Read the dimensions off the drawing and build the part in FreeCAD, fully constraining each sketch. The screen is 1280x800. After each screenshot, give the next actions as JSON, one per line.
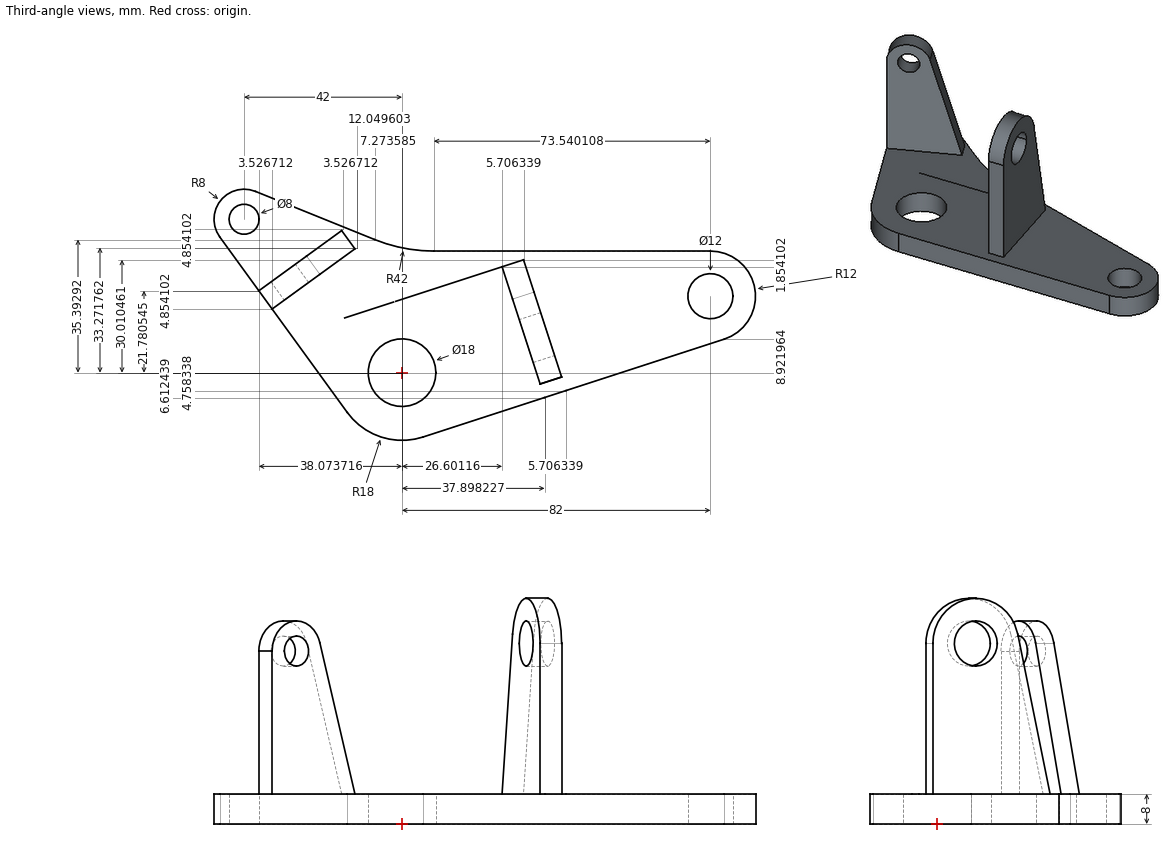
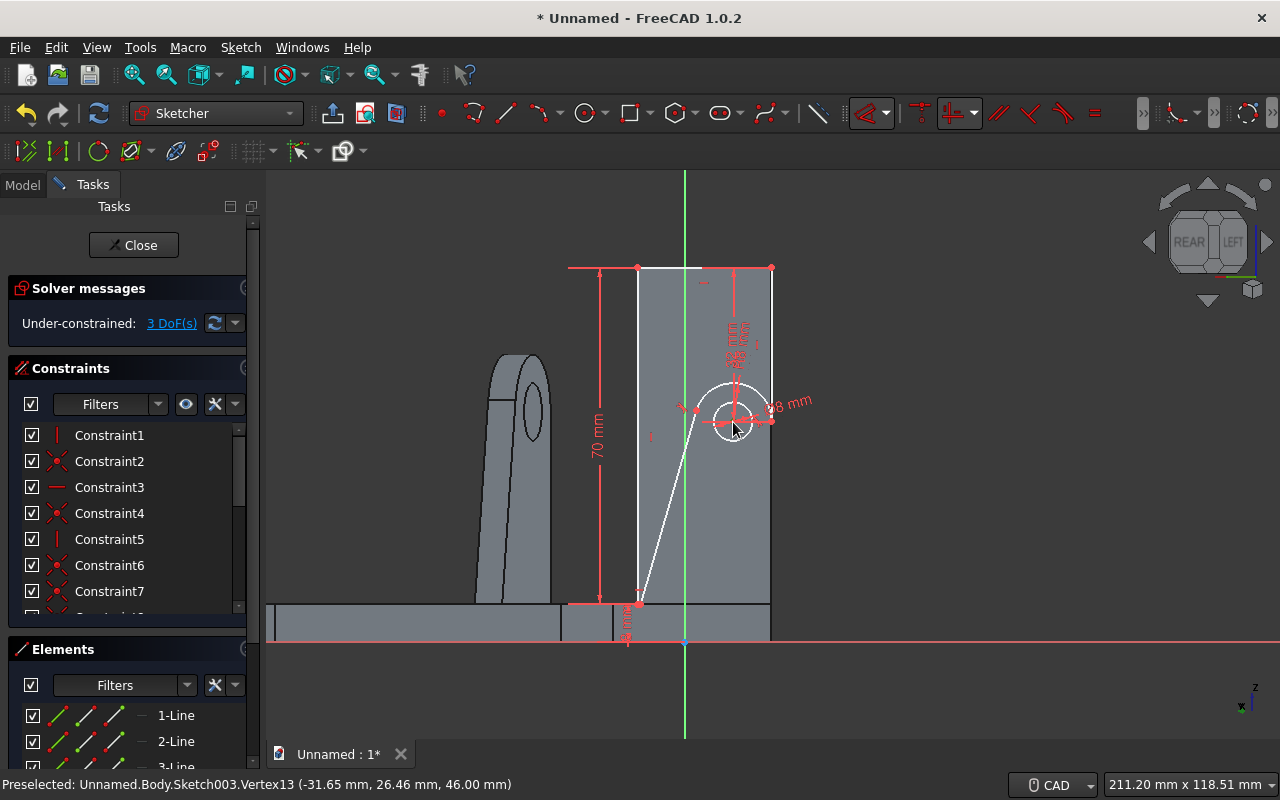
{"action": "key", "text": "l"}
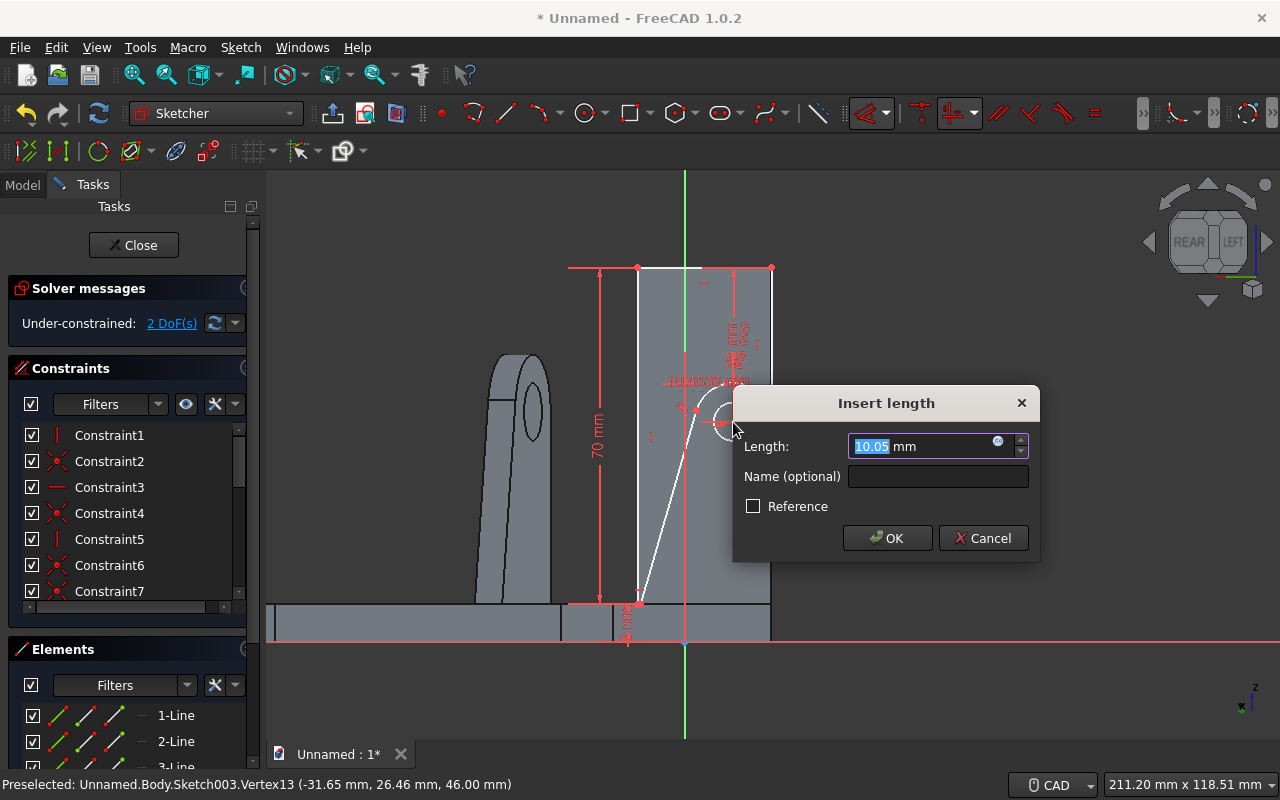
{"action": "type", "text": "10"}
{"action": "key", "text": "Return"}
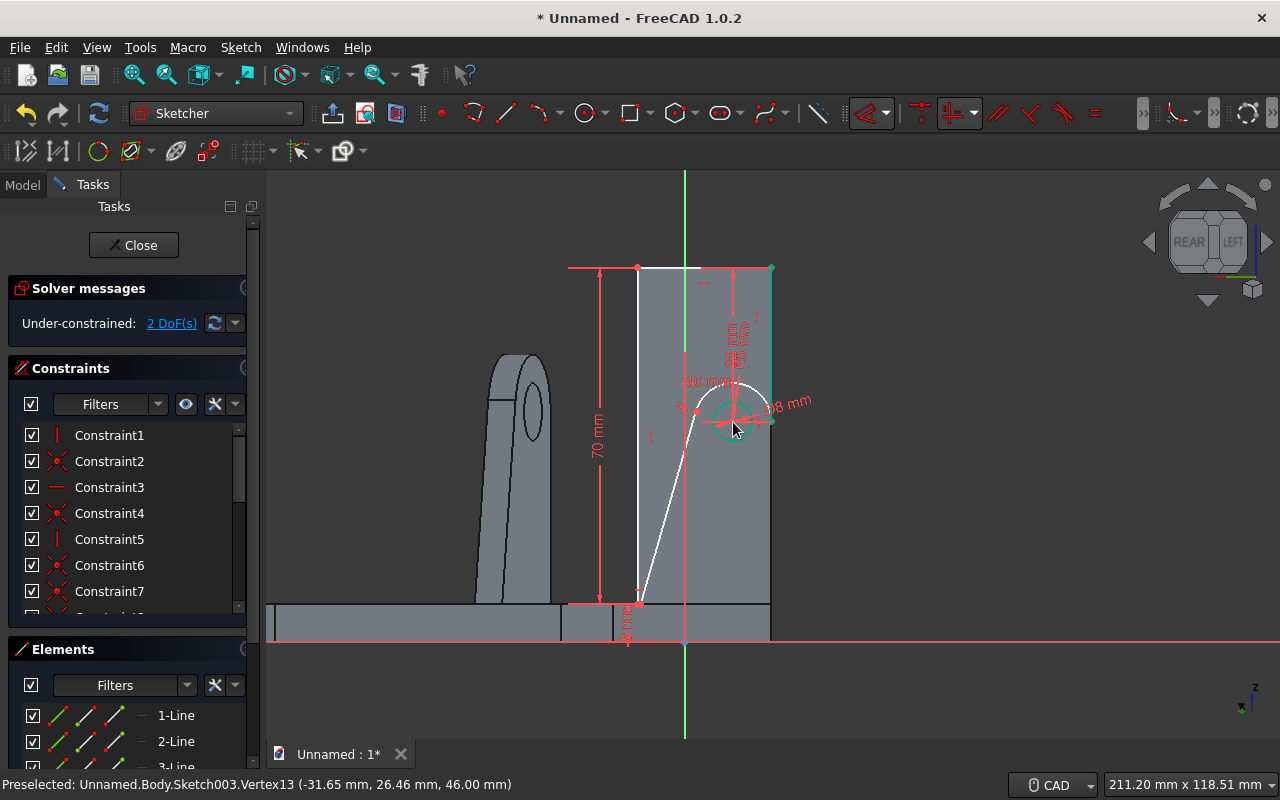
{"action": "scroll", "coordinate": [639, 604], "scroll_direction": "up", "scroll_amount": 14}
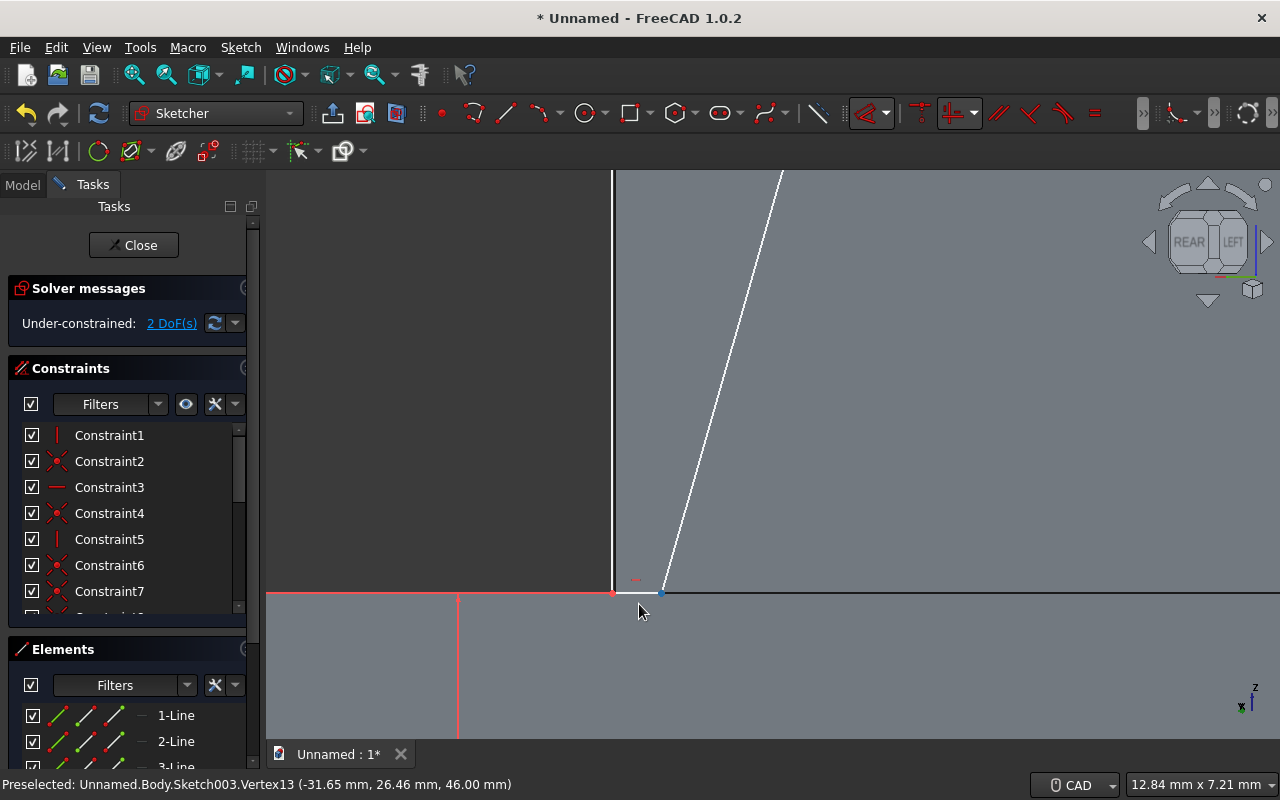
{"action": "left_click", "coordinate": [637, 593]}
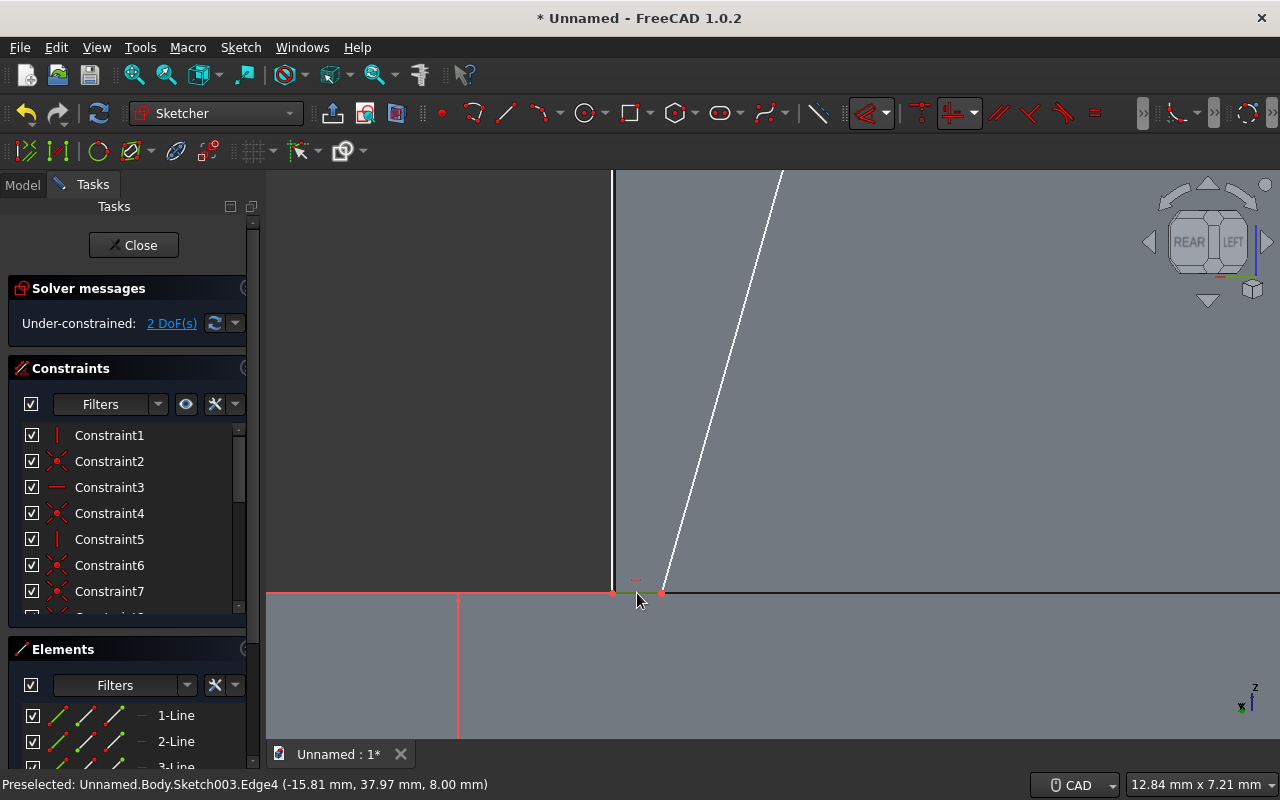
{"action": "key", "text": "l"}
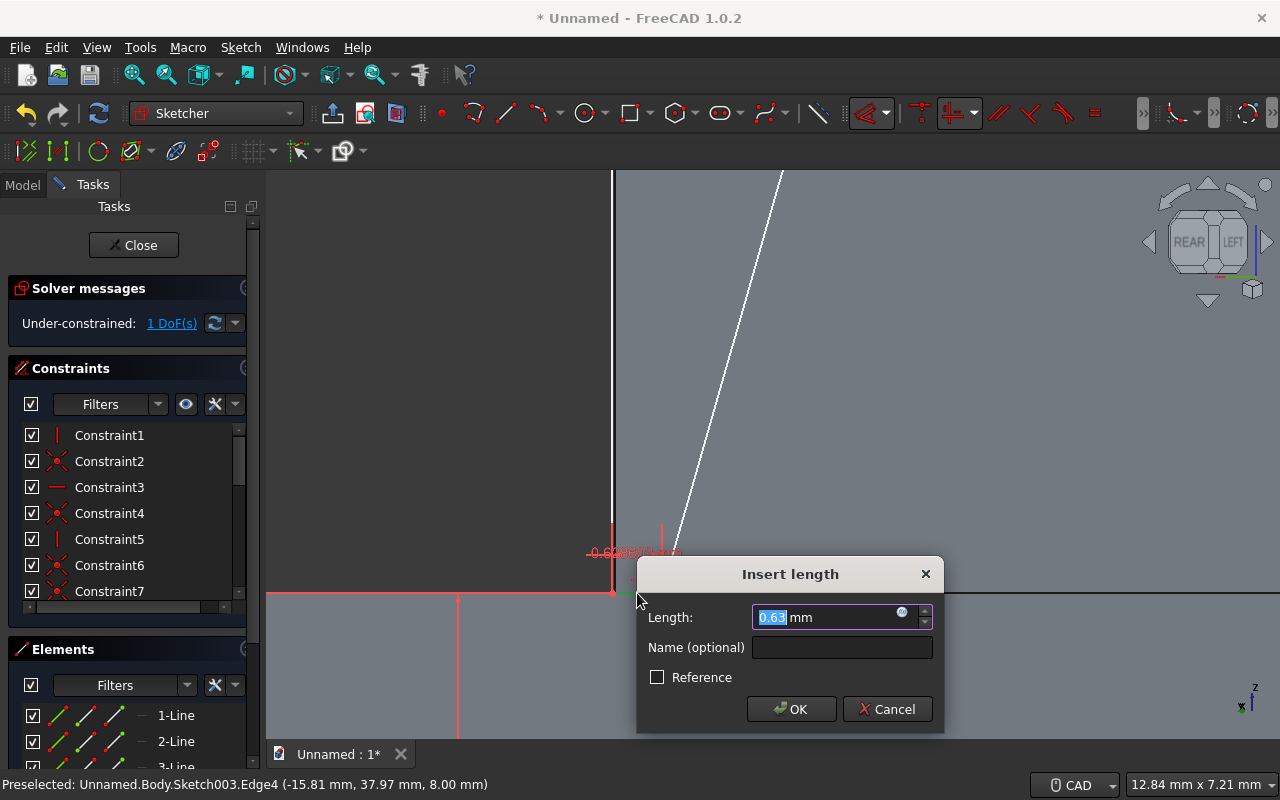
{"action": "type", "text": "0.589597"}
{"action": "key", "text": "Return"}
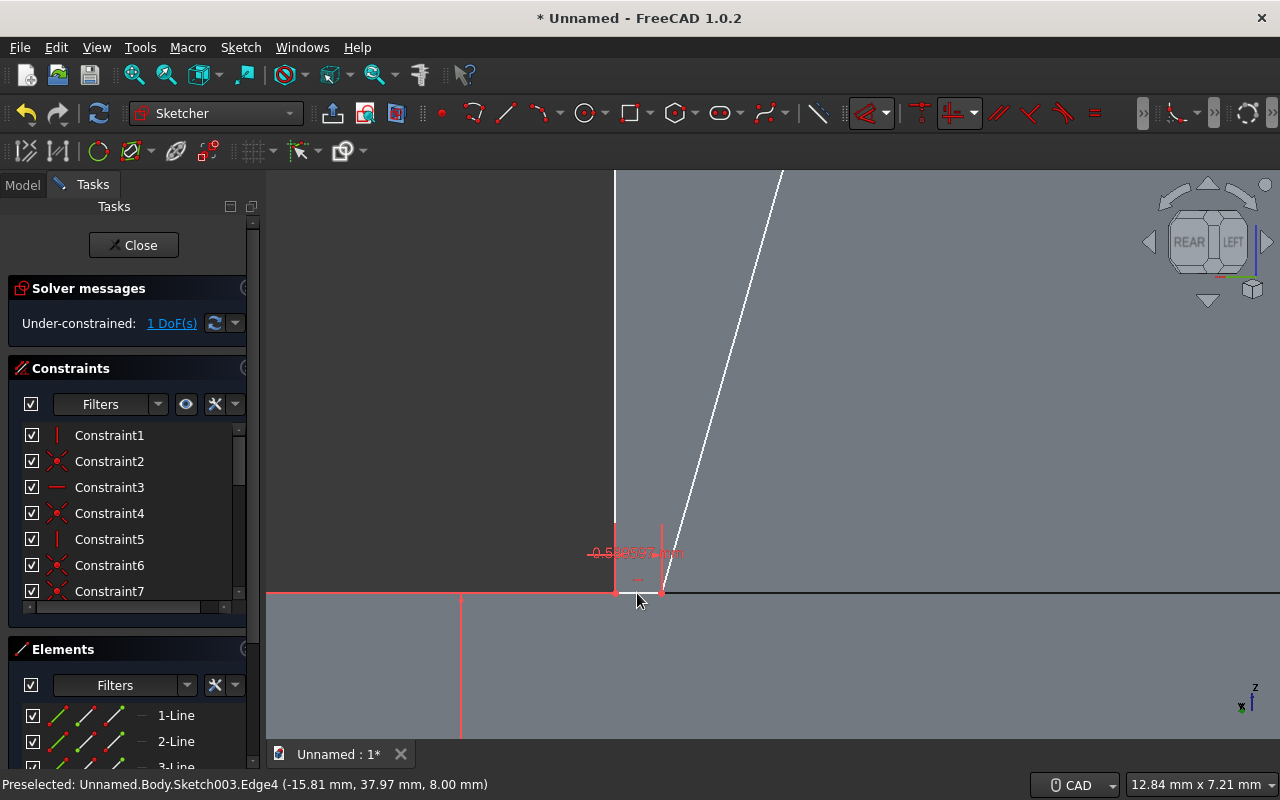
{"action": "scroll", "coordinate": [639, 604], "scroll_direction": "down", "scroll_amount": 14}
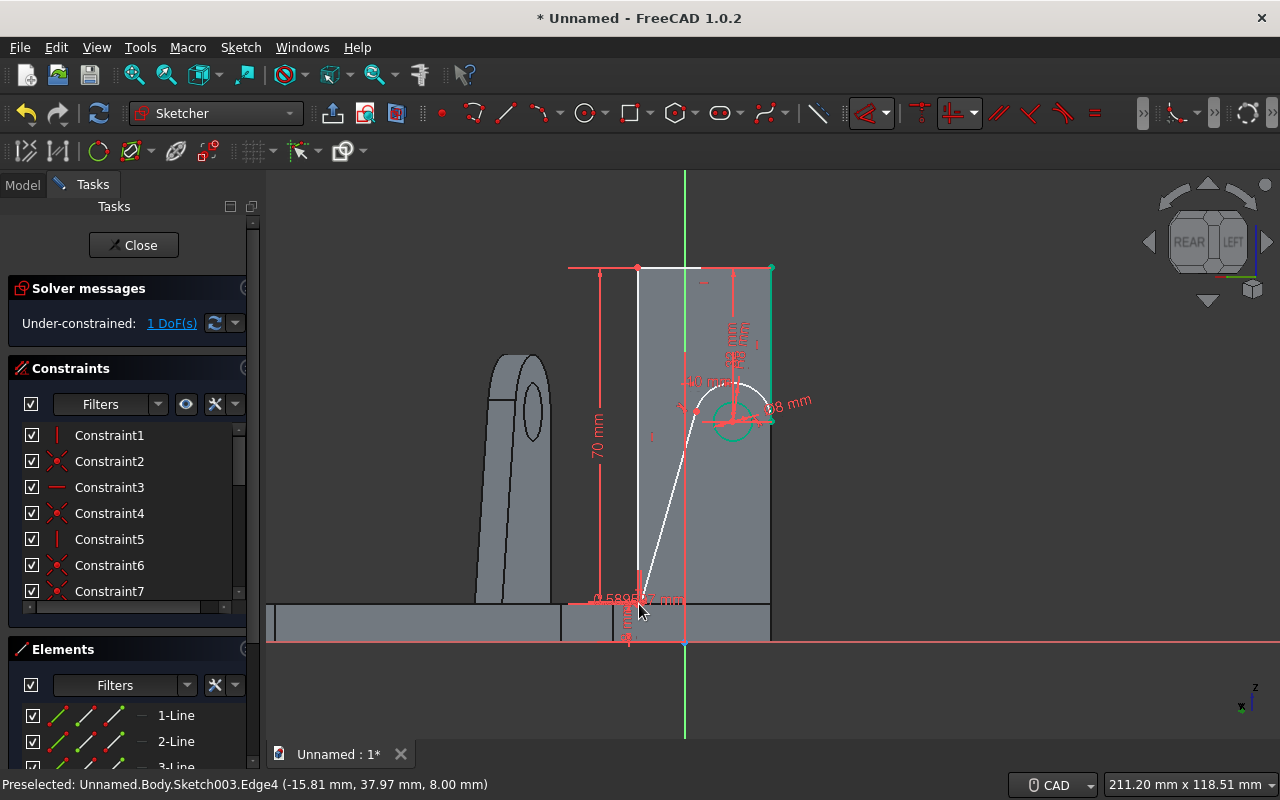
{"action": "left_click", "coordinate": [731, 268]}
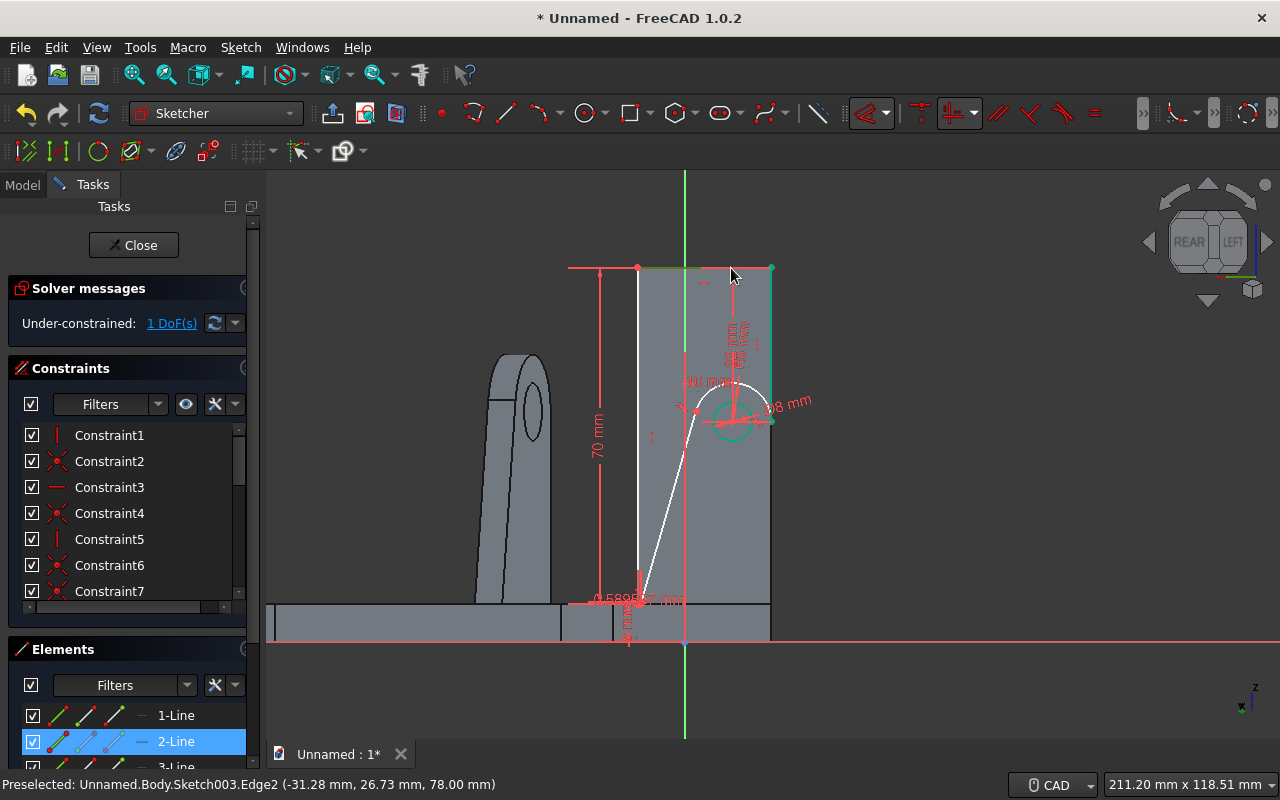
{"action": "key", "text": "l"}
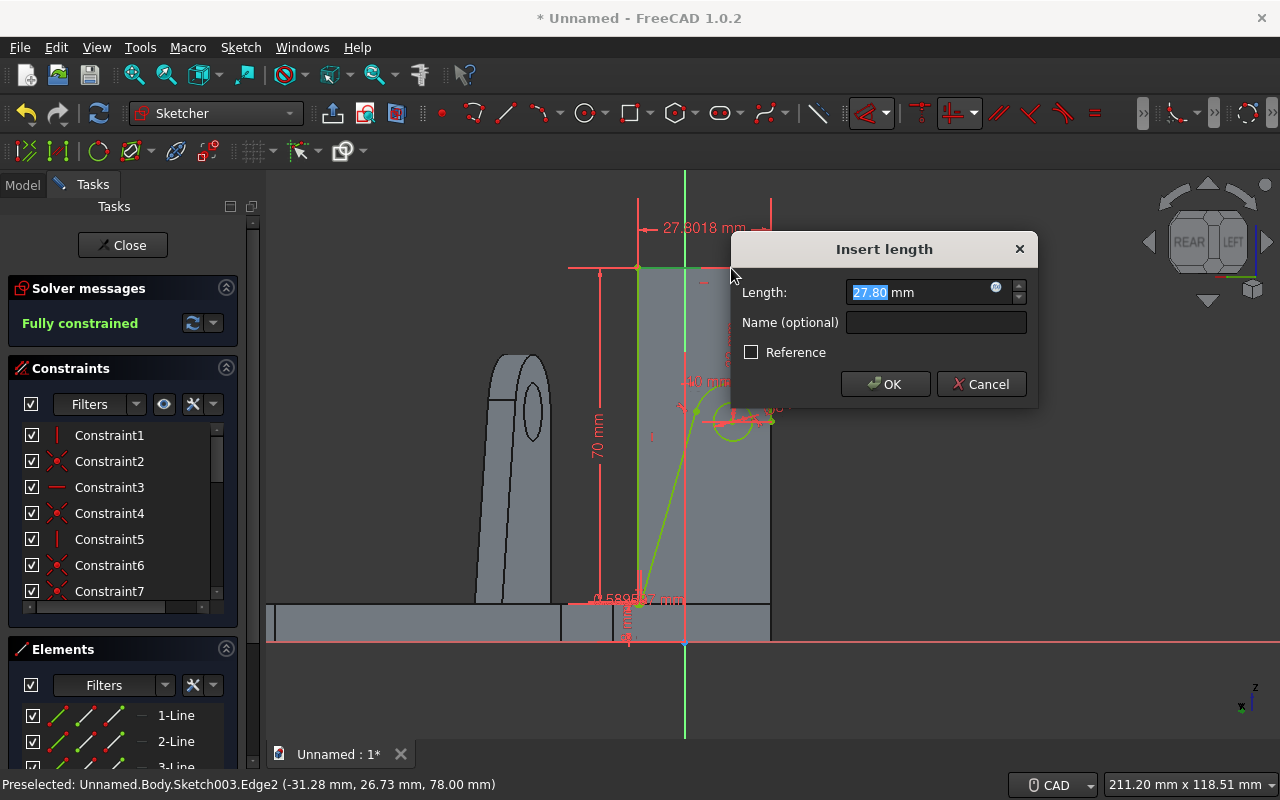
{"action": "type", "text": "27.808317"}
{"action": "key", "text": "Return"}